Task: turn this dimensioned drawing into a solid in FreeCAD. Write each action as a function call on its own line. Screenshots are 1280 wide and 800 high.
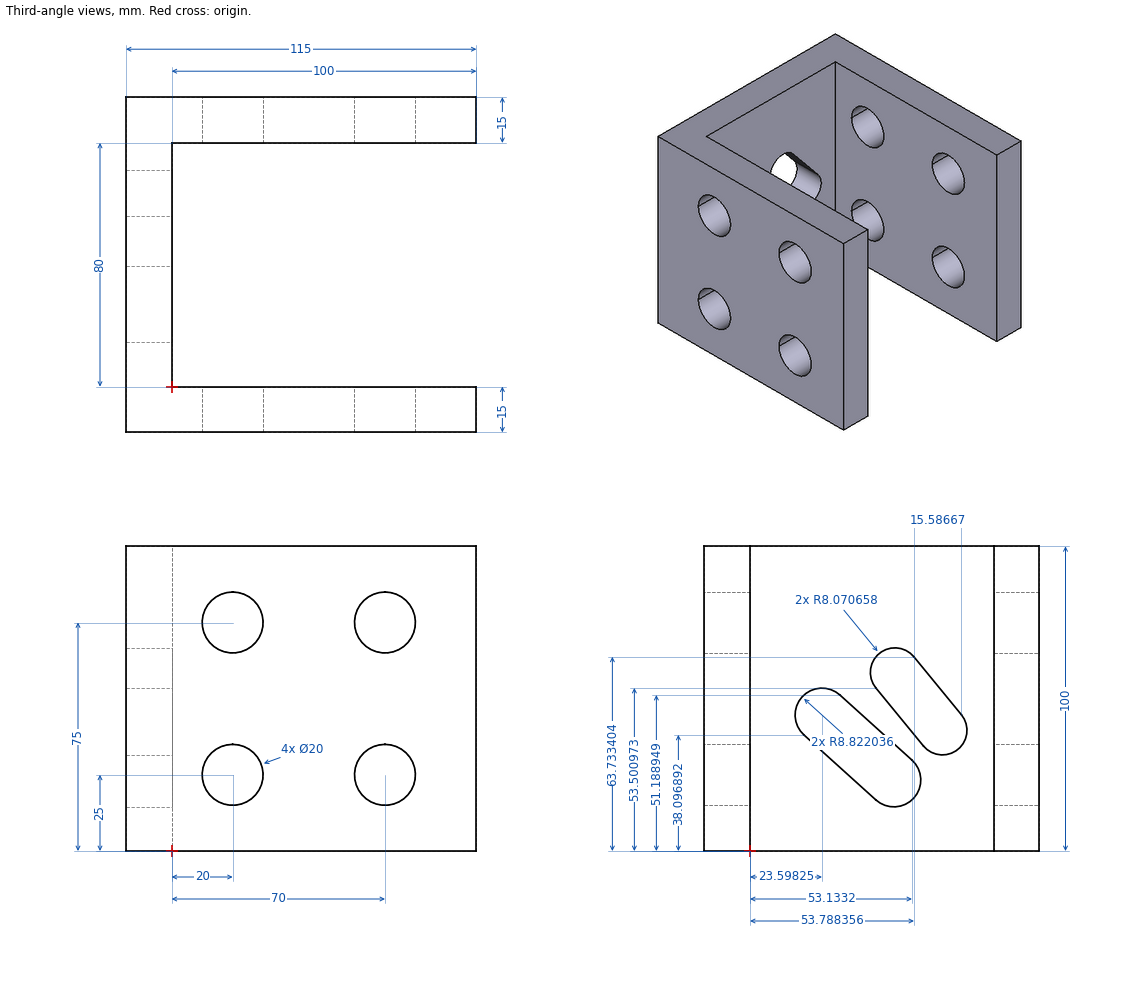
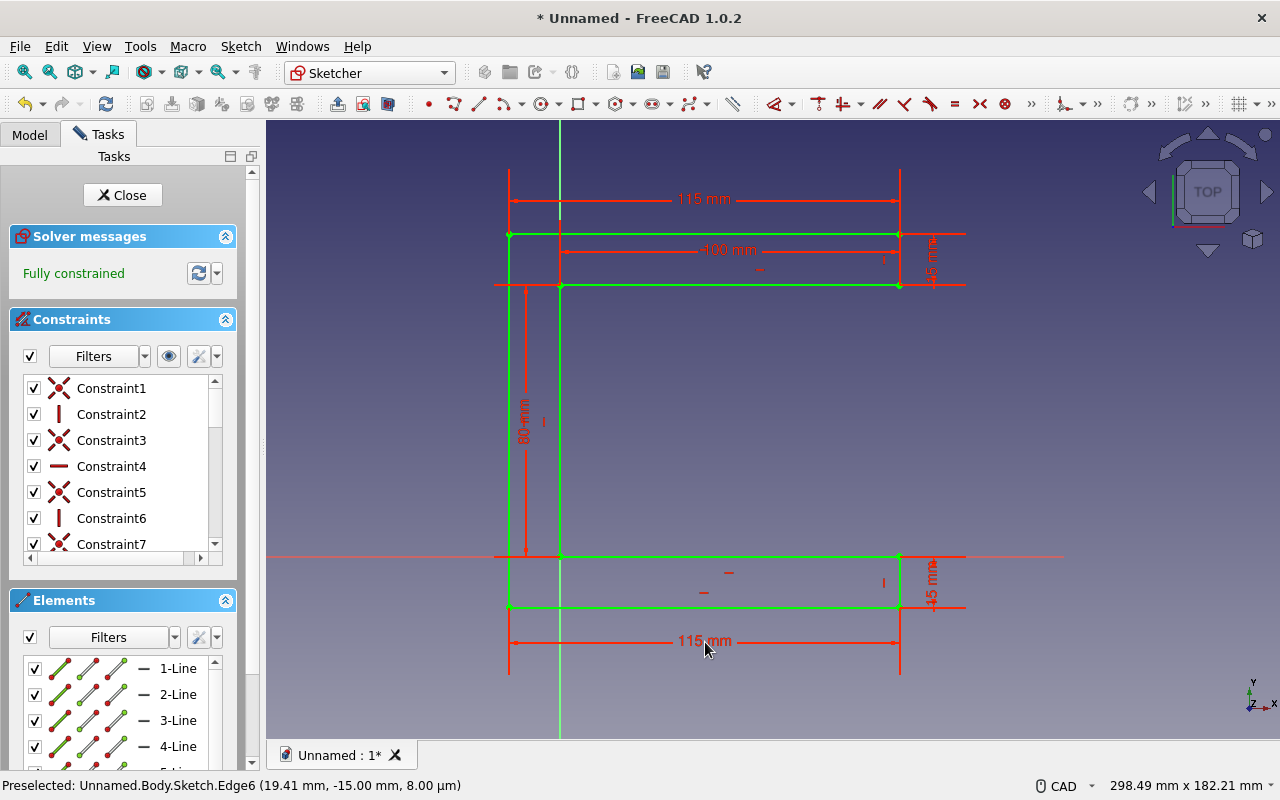
click(123, 195)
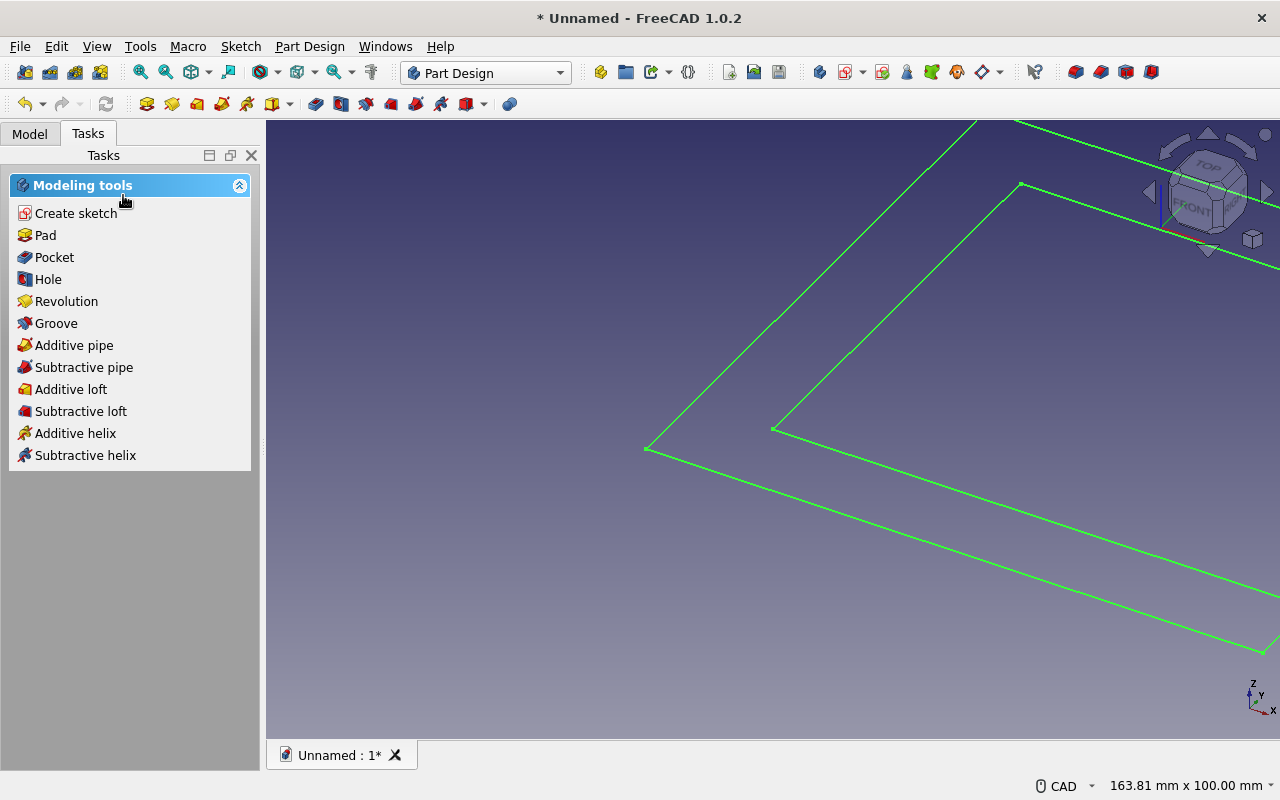
click(147, 104)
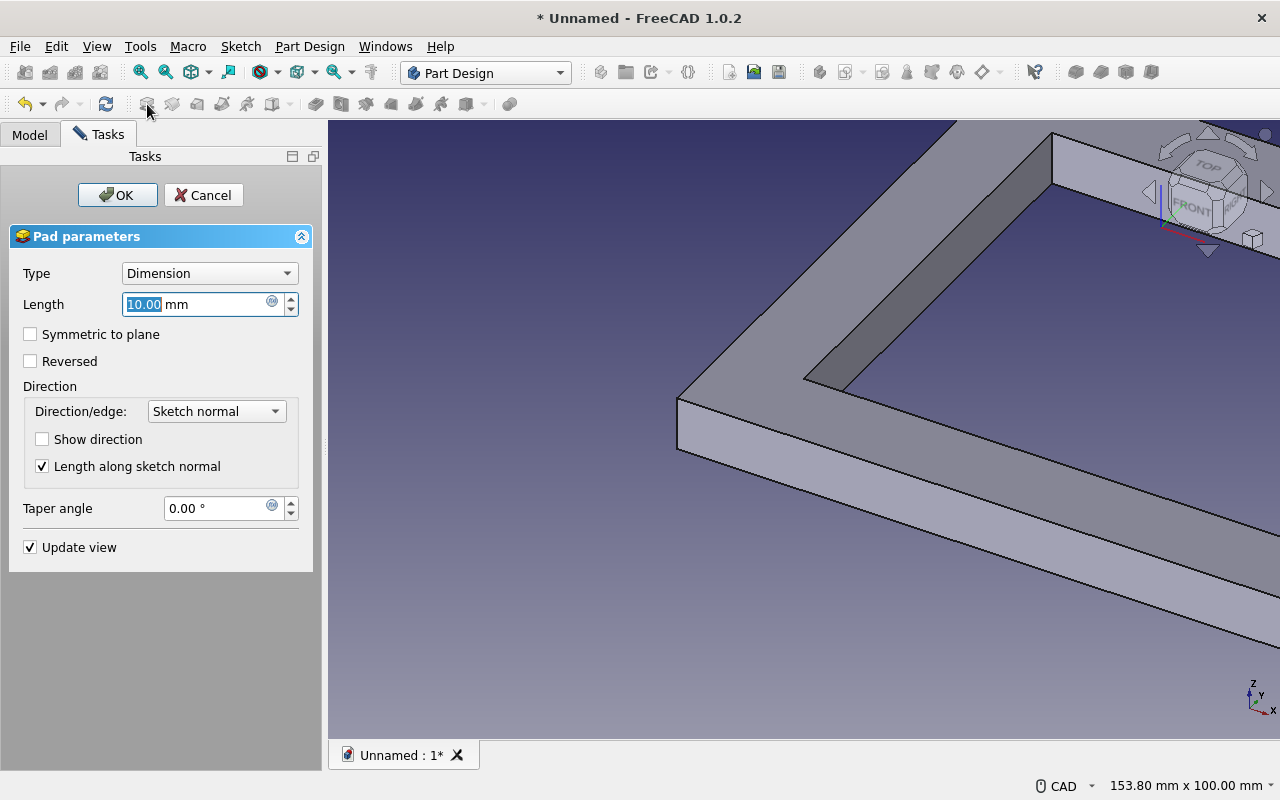
text(100)
key(Tab)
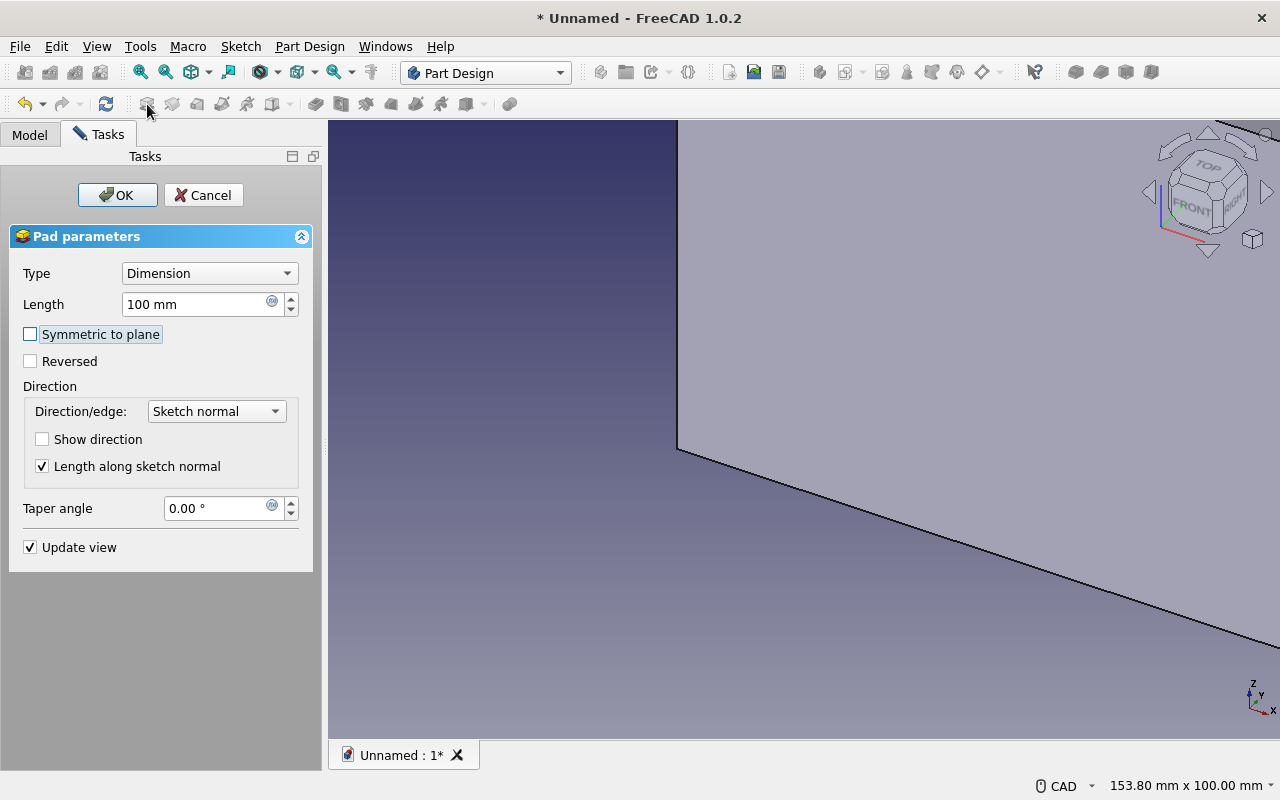
click(118, 195)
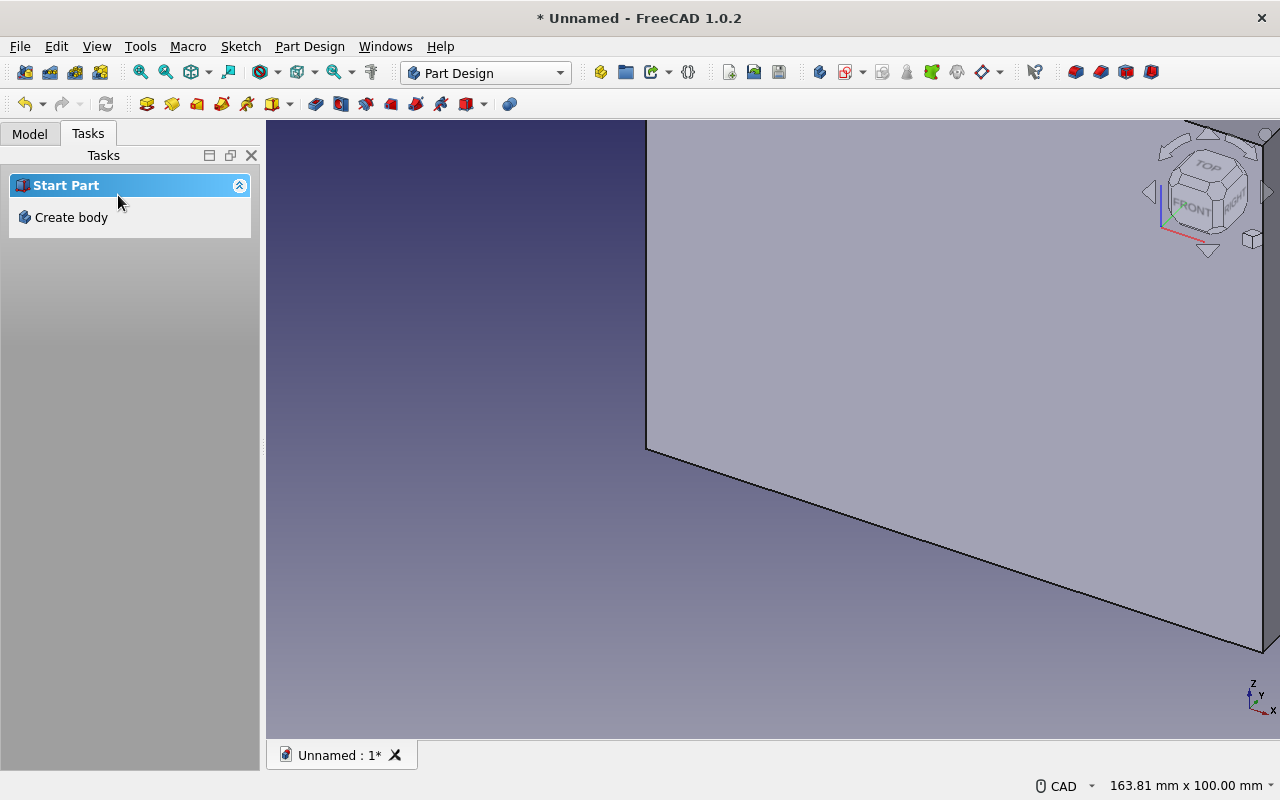
click(141, 72)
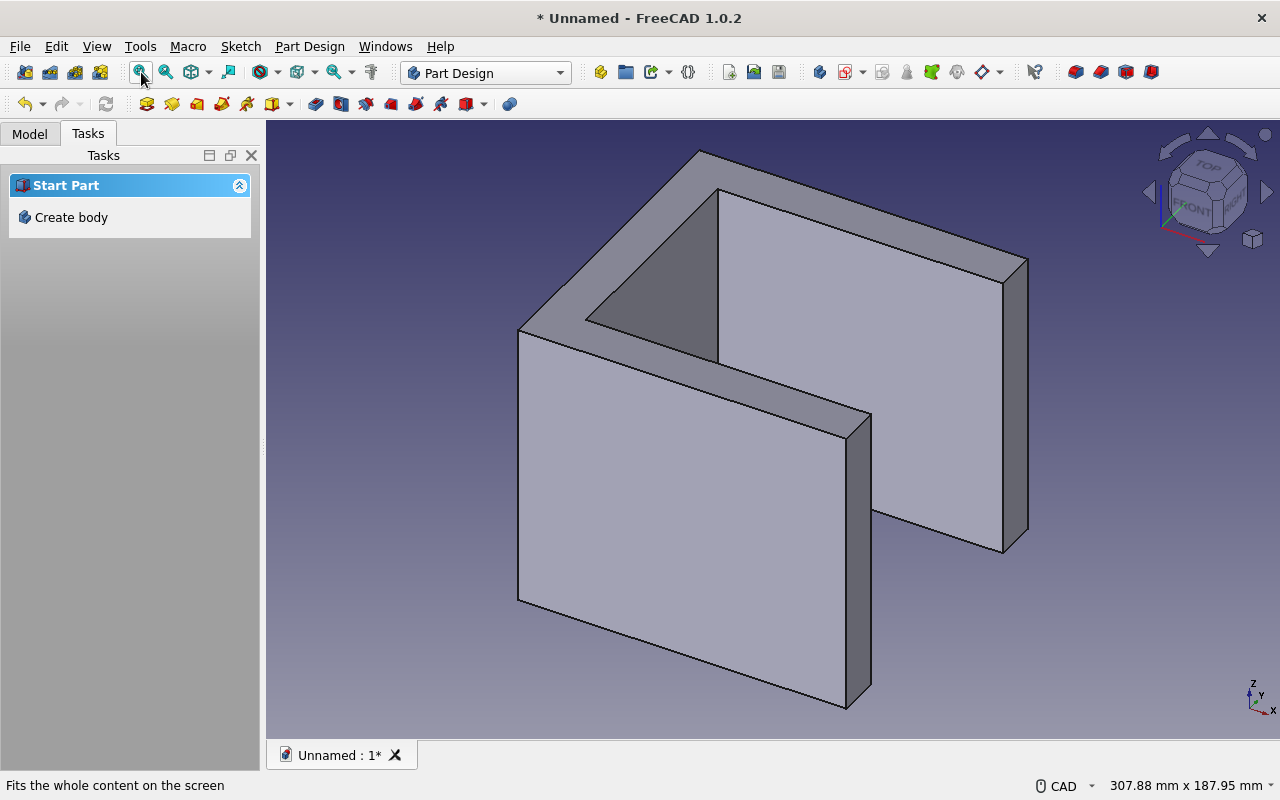
key(4)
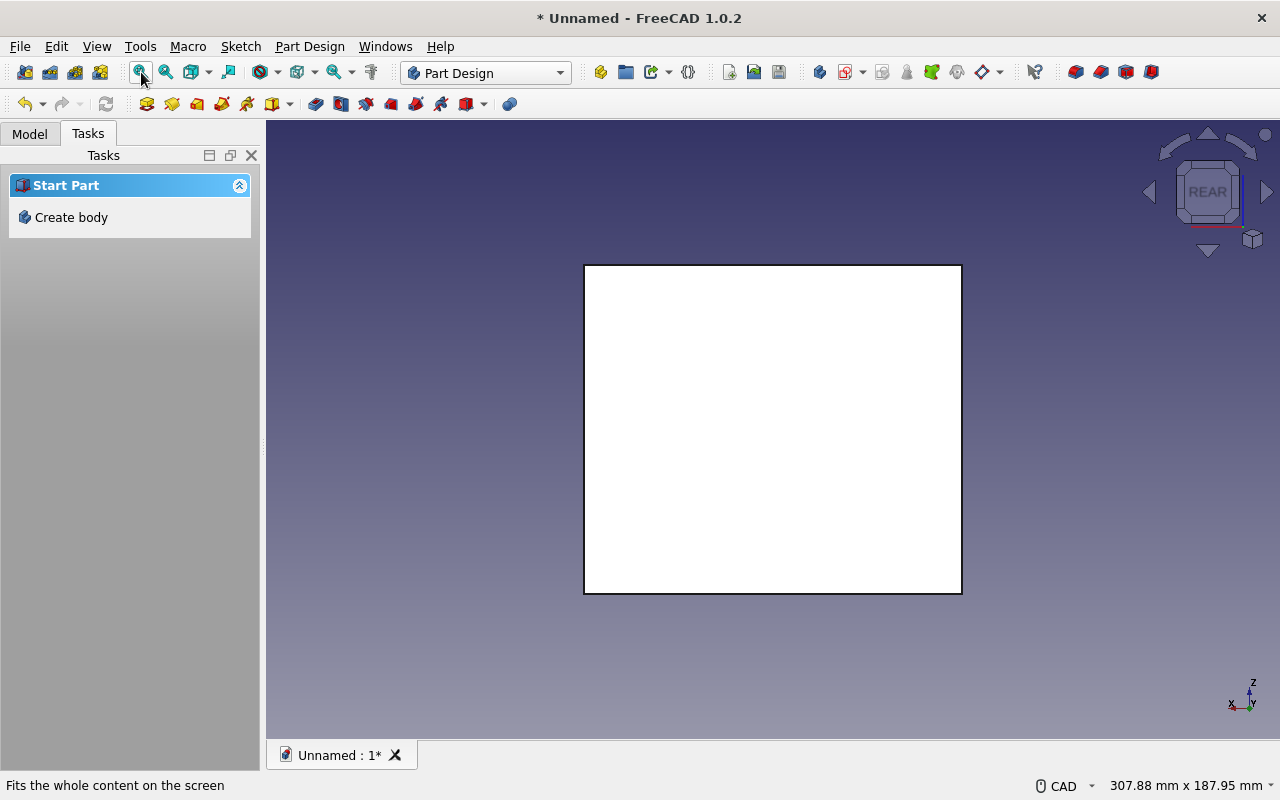
click(773, 429)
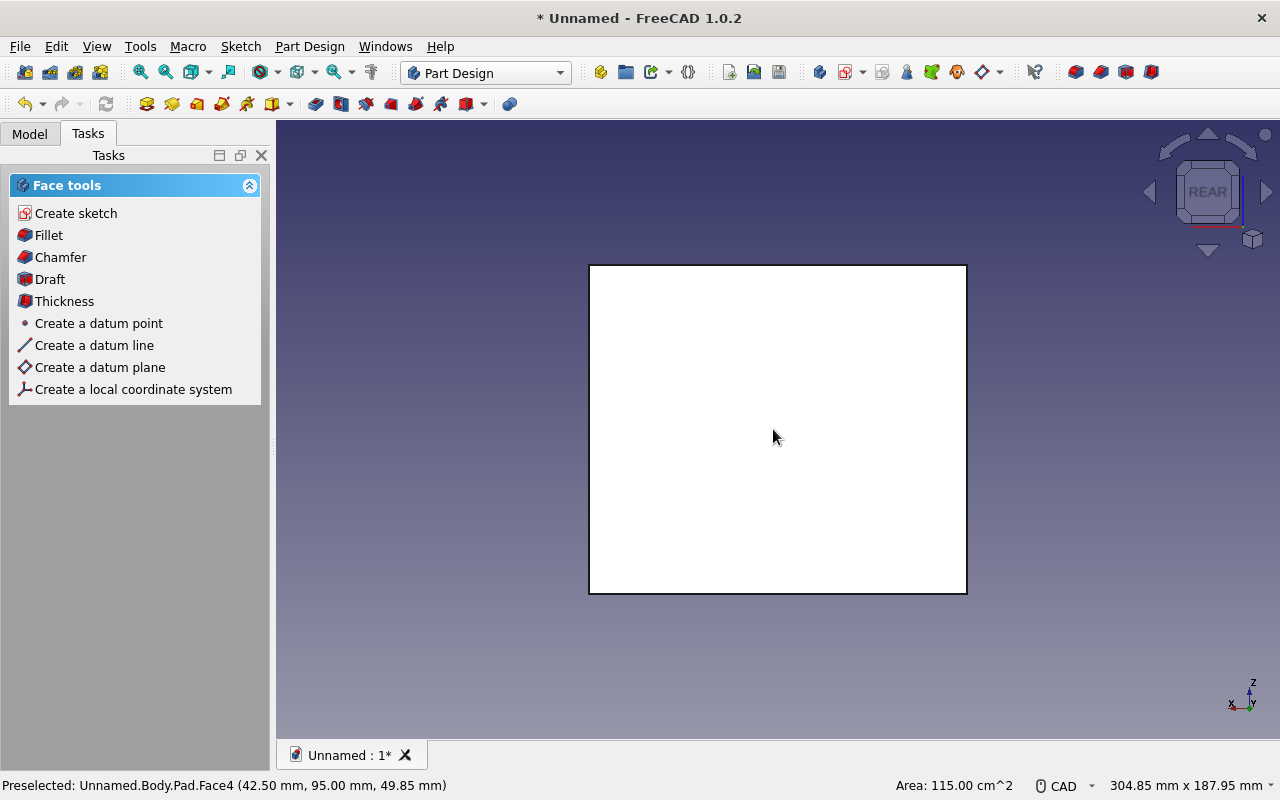
click(844, 72)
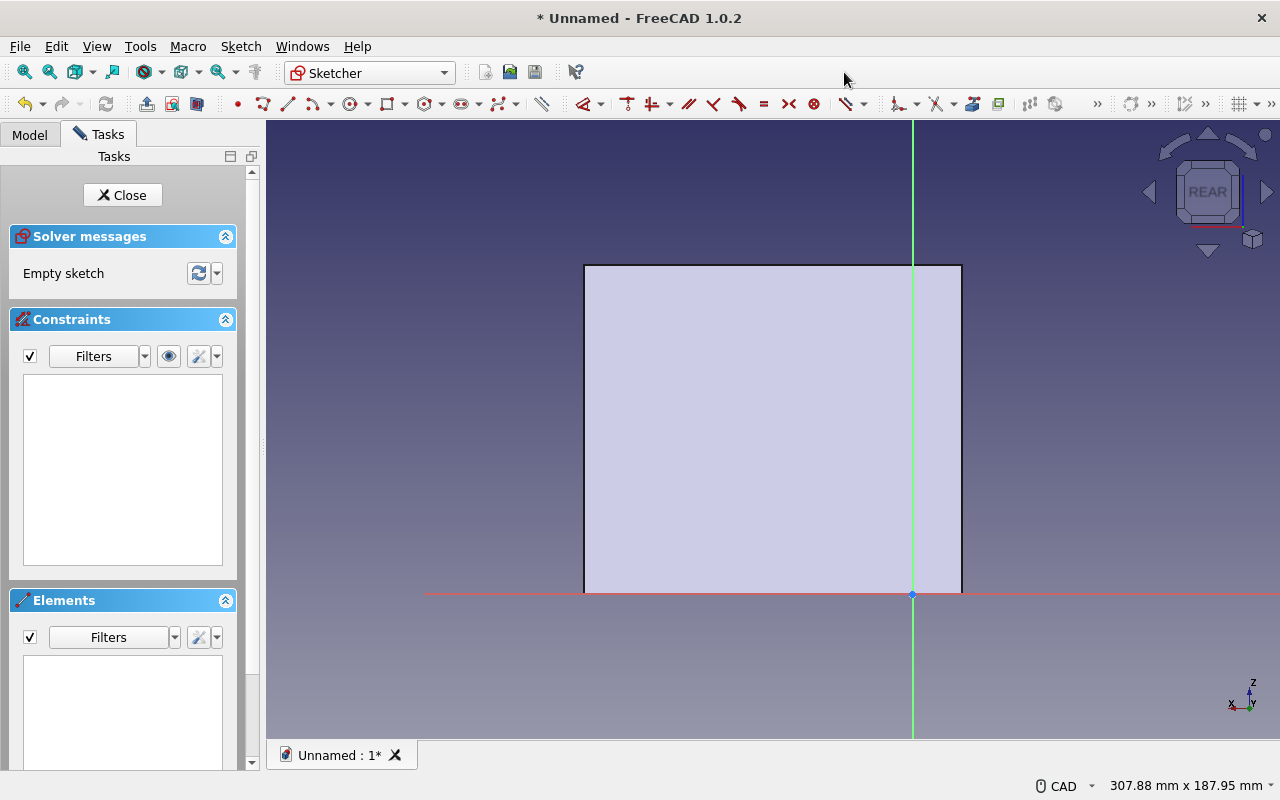
scroll(937, 504, up, 2)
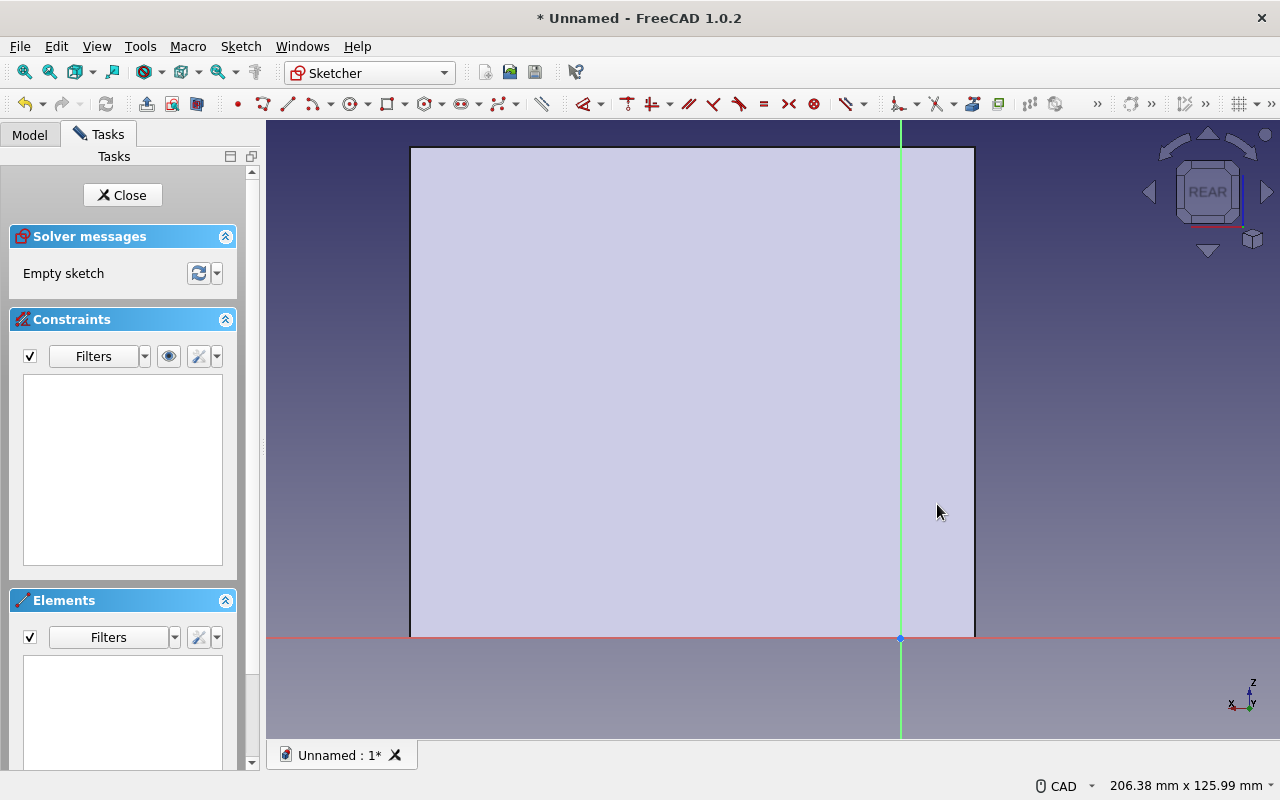
click(350, 104)